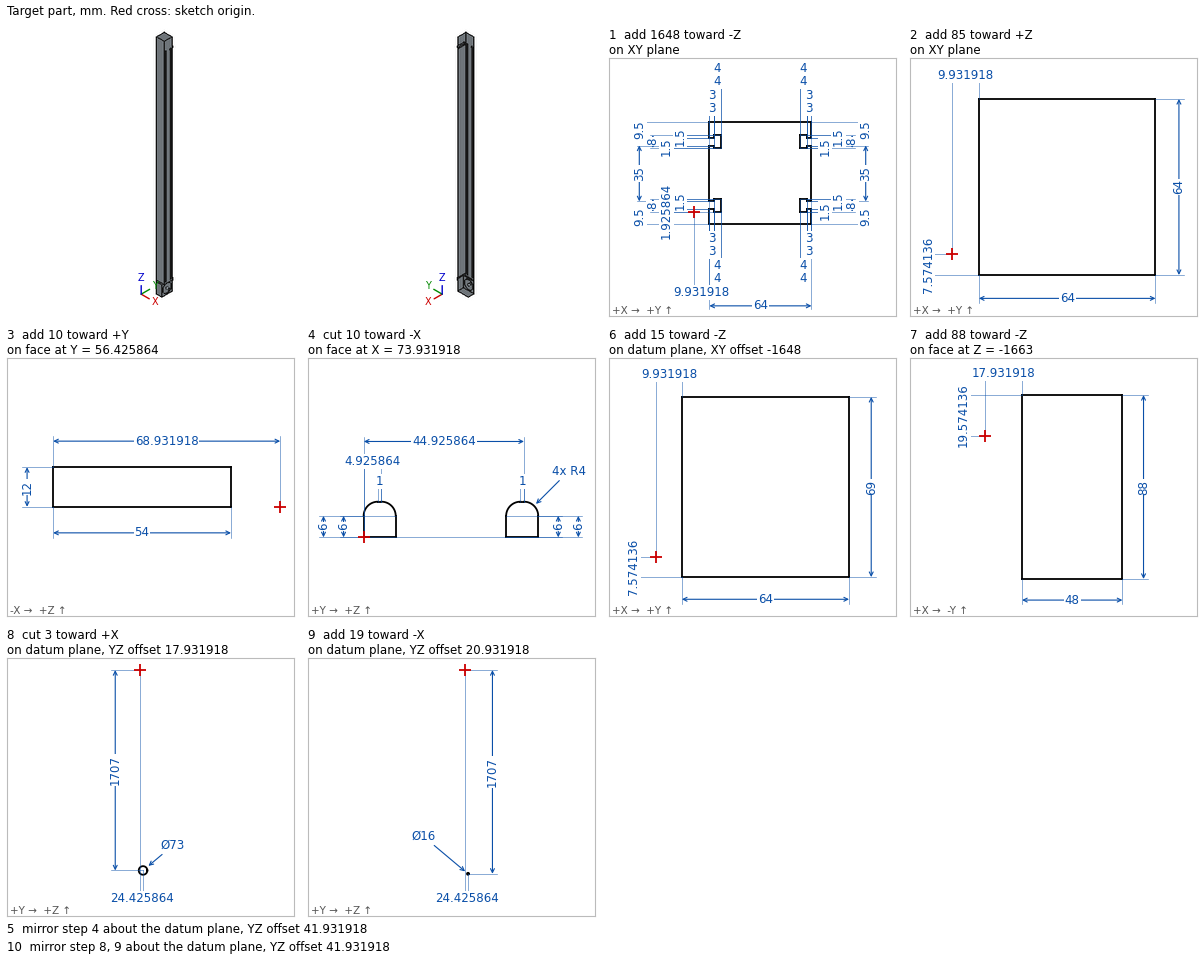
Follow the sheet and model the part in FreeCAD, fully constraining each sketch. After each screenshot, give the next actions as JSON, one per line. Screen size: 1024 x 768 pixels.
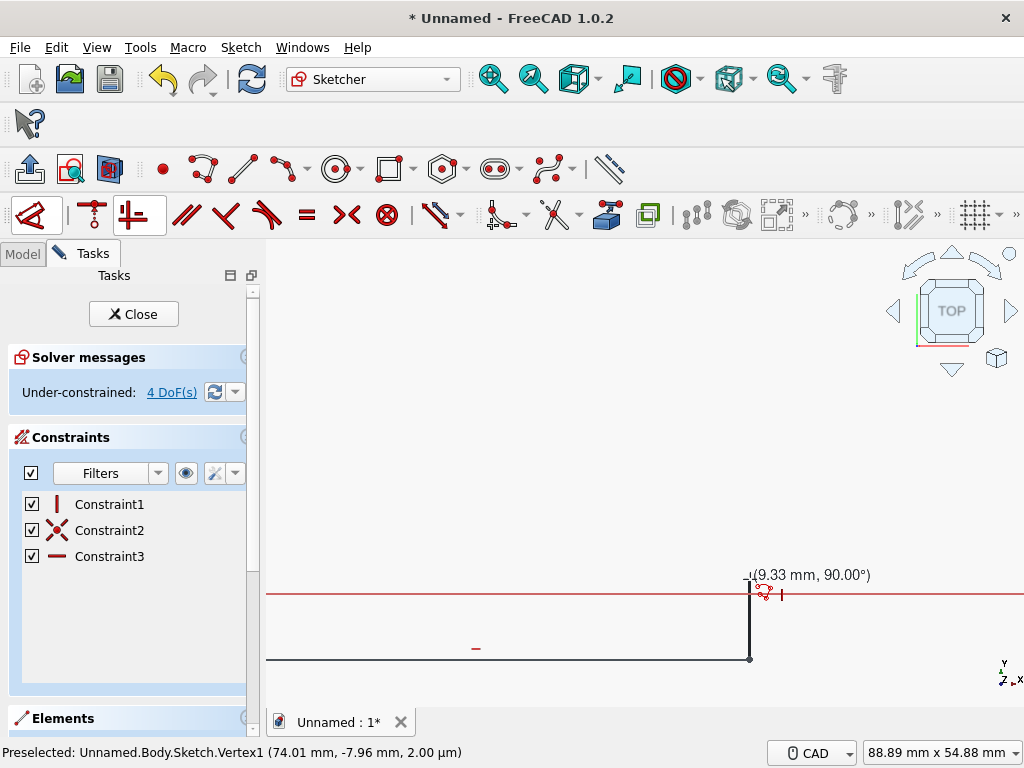
{"action": "left_click", "coordinate": [749, 578]}
{"action": "left_click", "coordinate": [723, 578]}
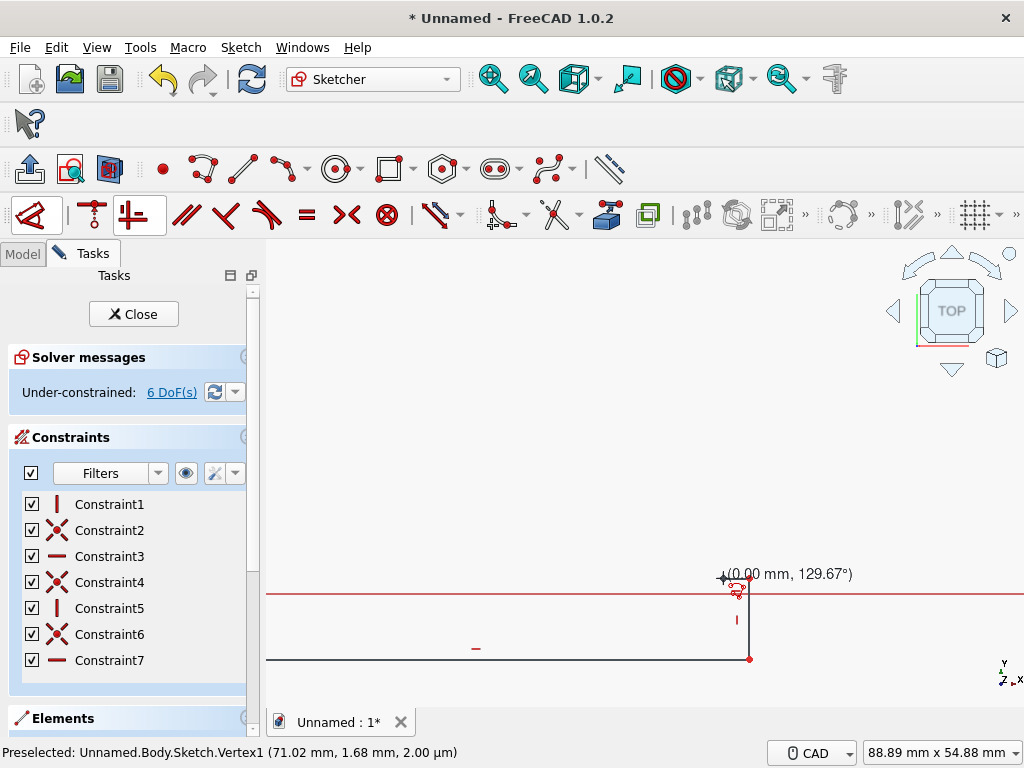
{"action": "scroll", "coordinate": [723, 591], "scroll_direction": "up", "scroll_amount": 8}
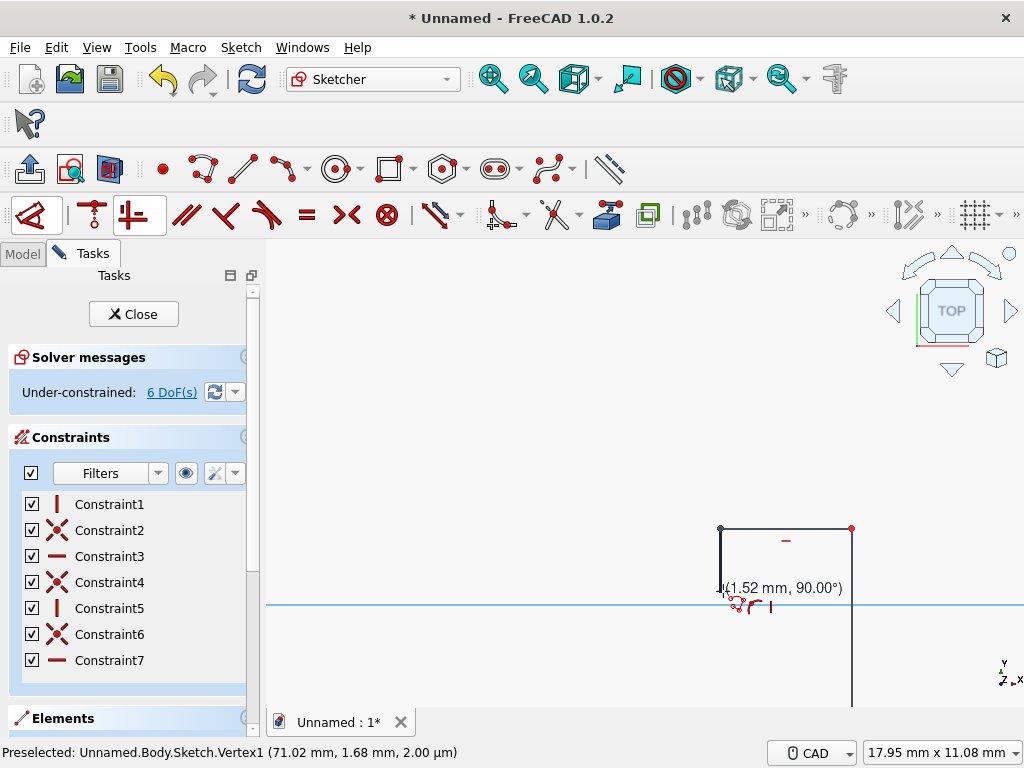
{"action": "left_click", "coordinate": [721, 587]}
{"action": "left_click", "coordinate": [553, 587]}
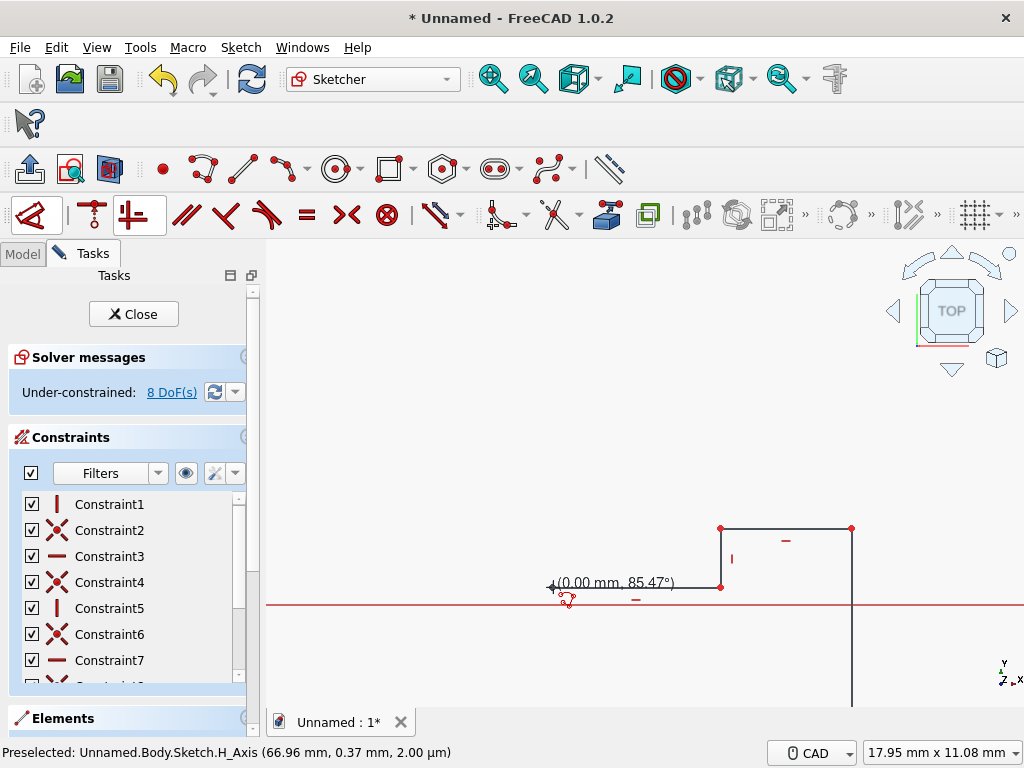
{"action": "scroll", "coordinate": [737, 585], "scroll_direction": "down", "scroll_amount": 11}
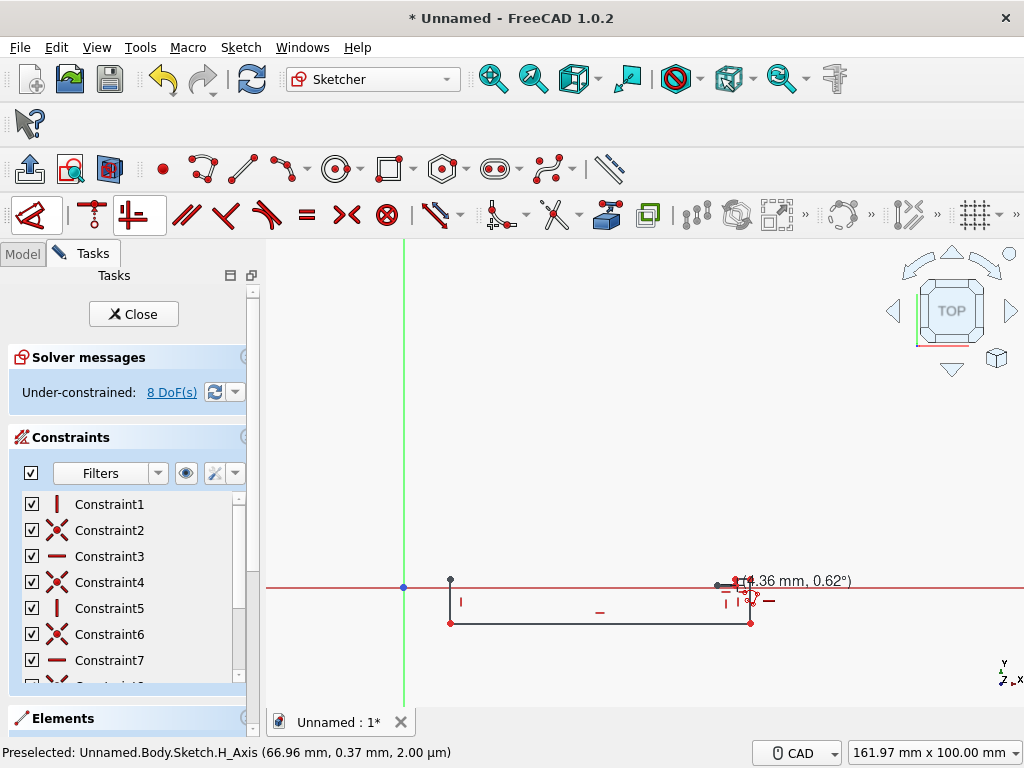
{"action": "left_click", "coordinate": [717, 548]}
{"action": "left_click", "coordinate": [736, 548]}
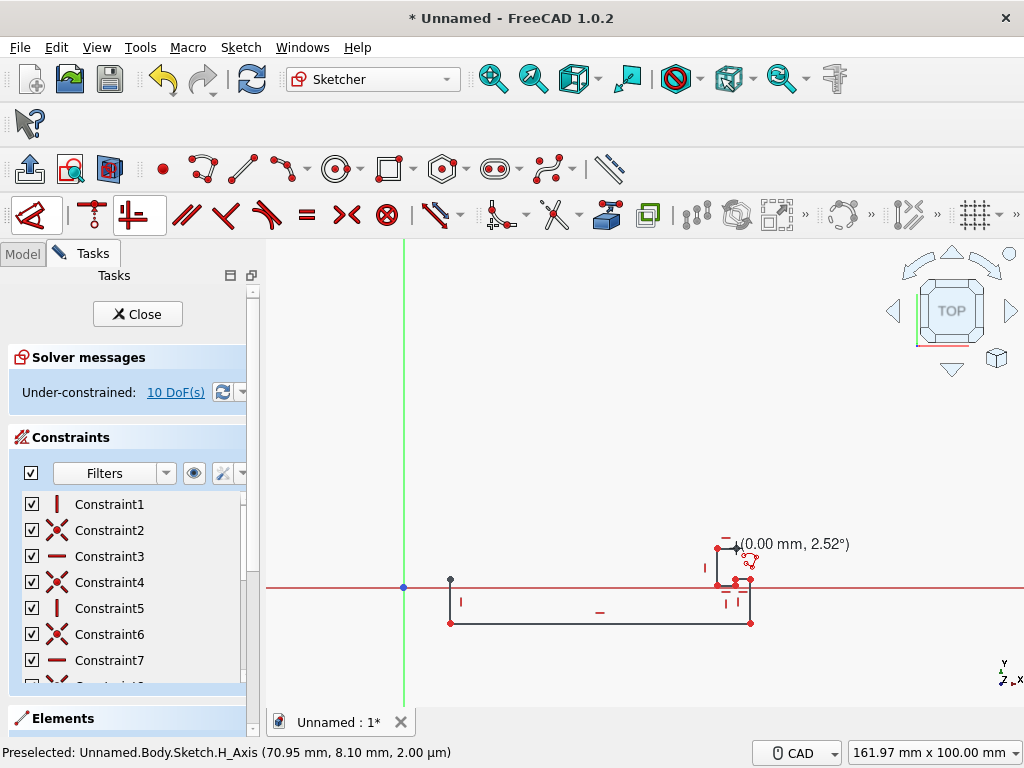
{"action": "scroll", "coordinate": [736, 555], "scroll_direction": "up", "scroll_amount": 5}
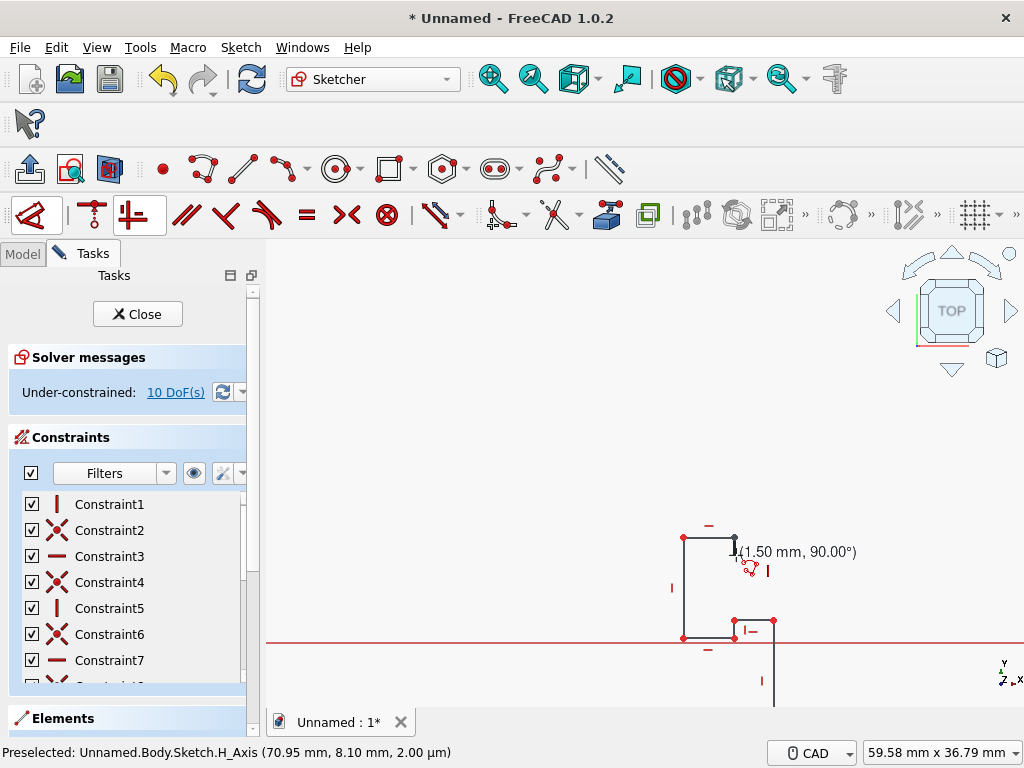
{"action": "left_click", "coordinate": [735, 555]}
{"action": "left_click", "coordinate": [773, 555]}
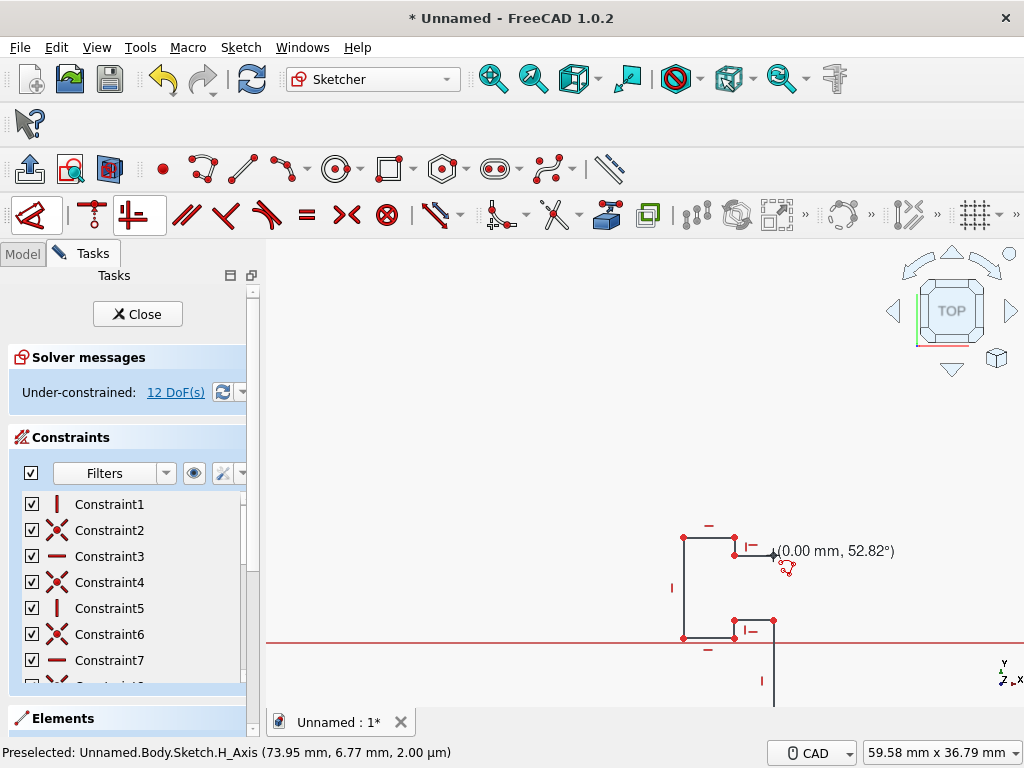
{"action": "scroll", "coordinate": [736, 555], "scroll_direction": "down", "scroll_amount": 5}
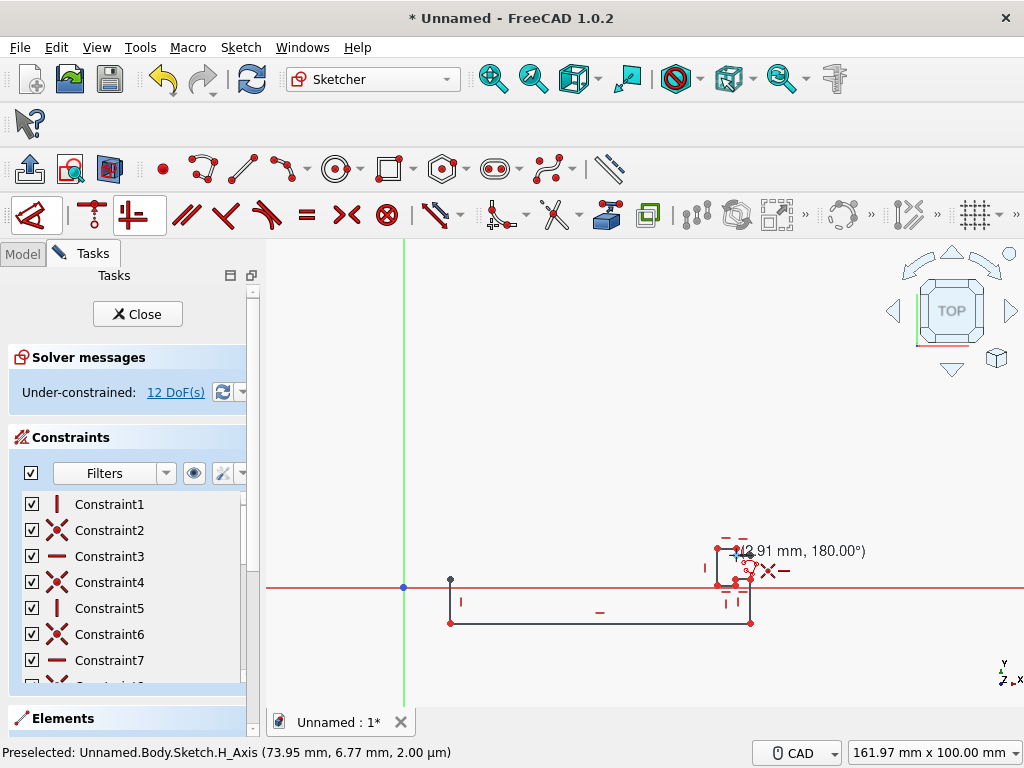
{"action": "left_click", "coordinate": [750, 392]}
{"action": "left_click", "coordinate": [736, 392]}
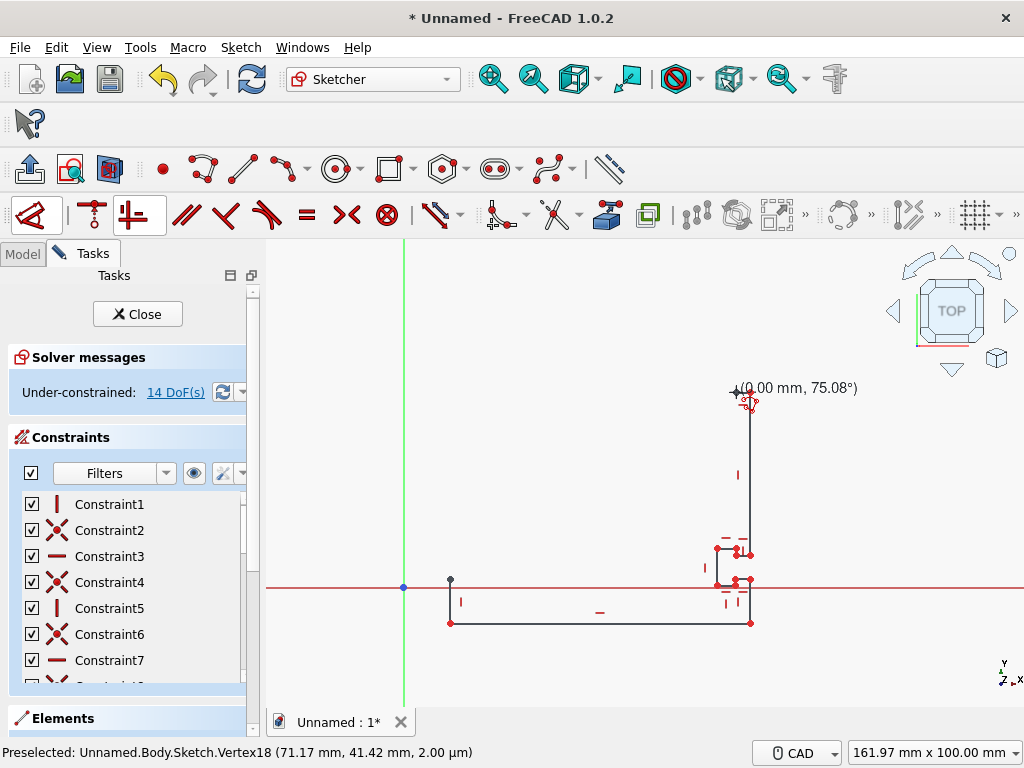
{"action": "scroll", "coordinate": [736, 399], "scroll_direction": "up", "scroll_amount": 5}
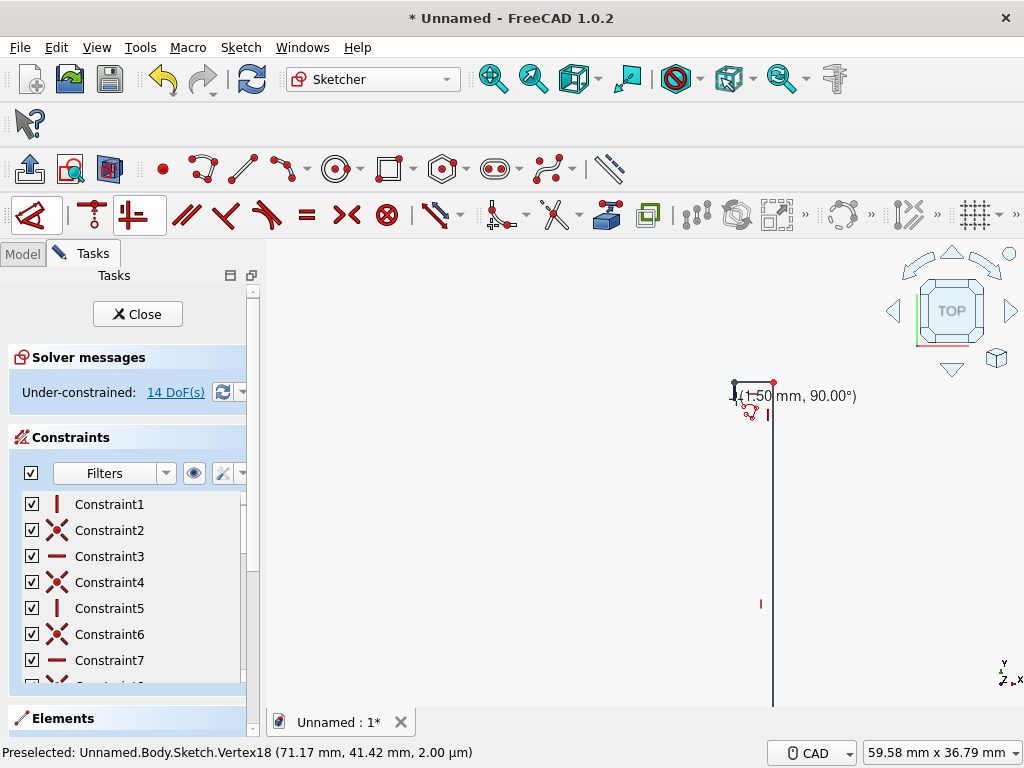
{"action": "left_click", "coordinate": [735, 397]}
{"action": "left_click", "coordinate": [684, 397]}
{"action": "left_click", "coordinate": [684, 296]}
{"action": "left_click", "coordinate": [735, 296]}
{"action": "left_click", "coordinate": [735, 315]}
{"action": "left_click", "coordinate": [773, 315]}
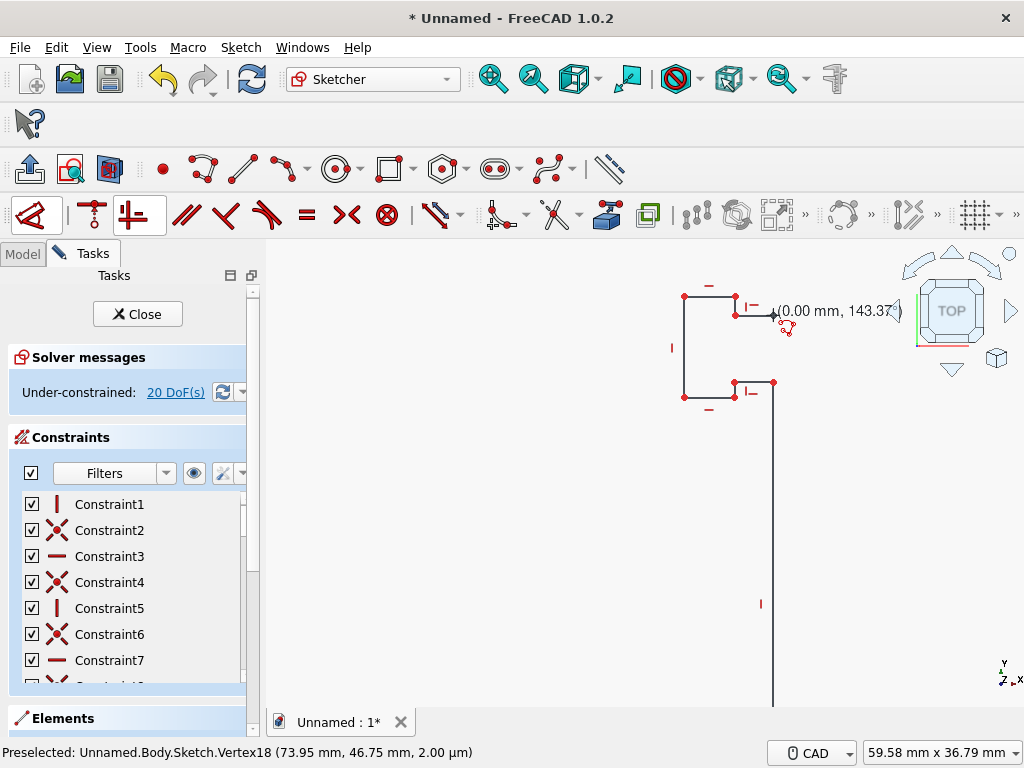
{"action": "scroll", "coordinate": [736, 399], "scroll_direction": "down", "scroll_amount": 5}